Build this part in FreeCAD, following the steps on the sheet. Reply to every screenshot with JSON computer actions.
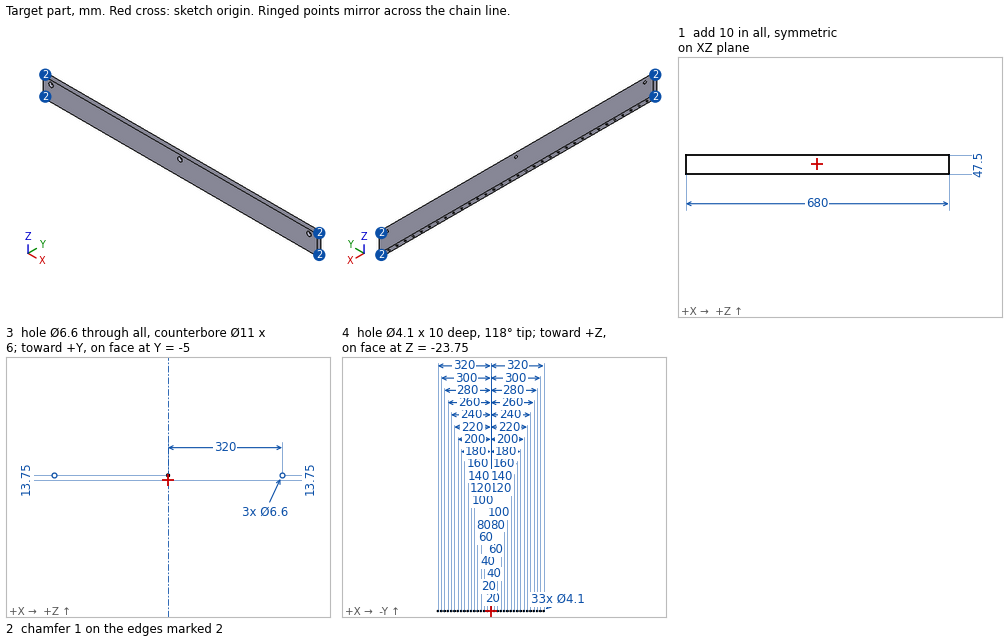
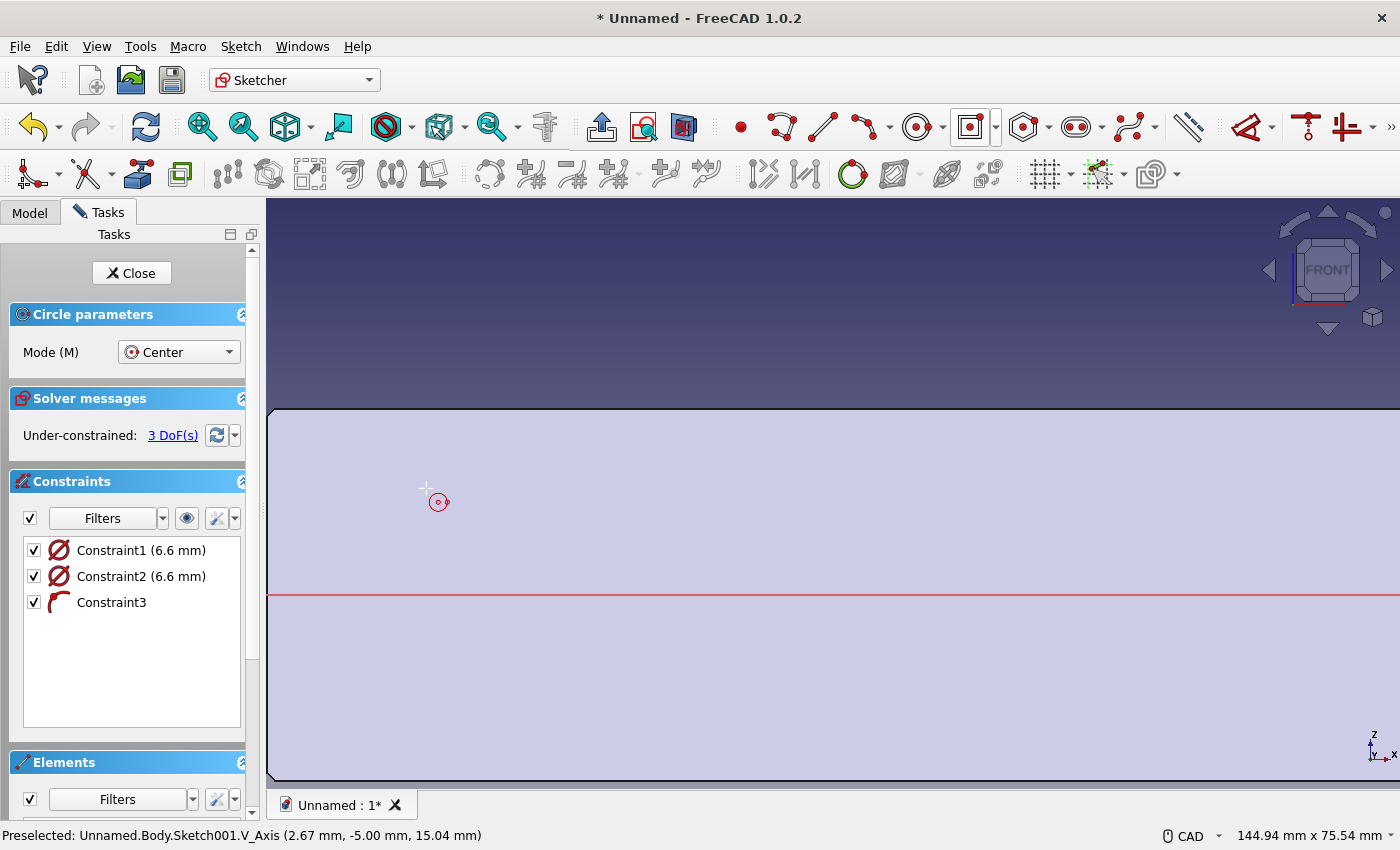
{"action": "scroll", "coordinate": [426, 488], "scroll_direction": "down", "scroll_amount": 10}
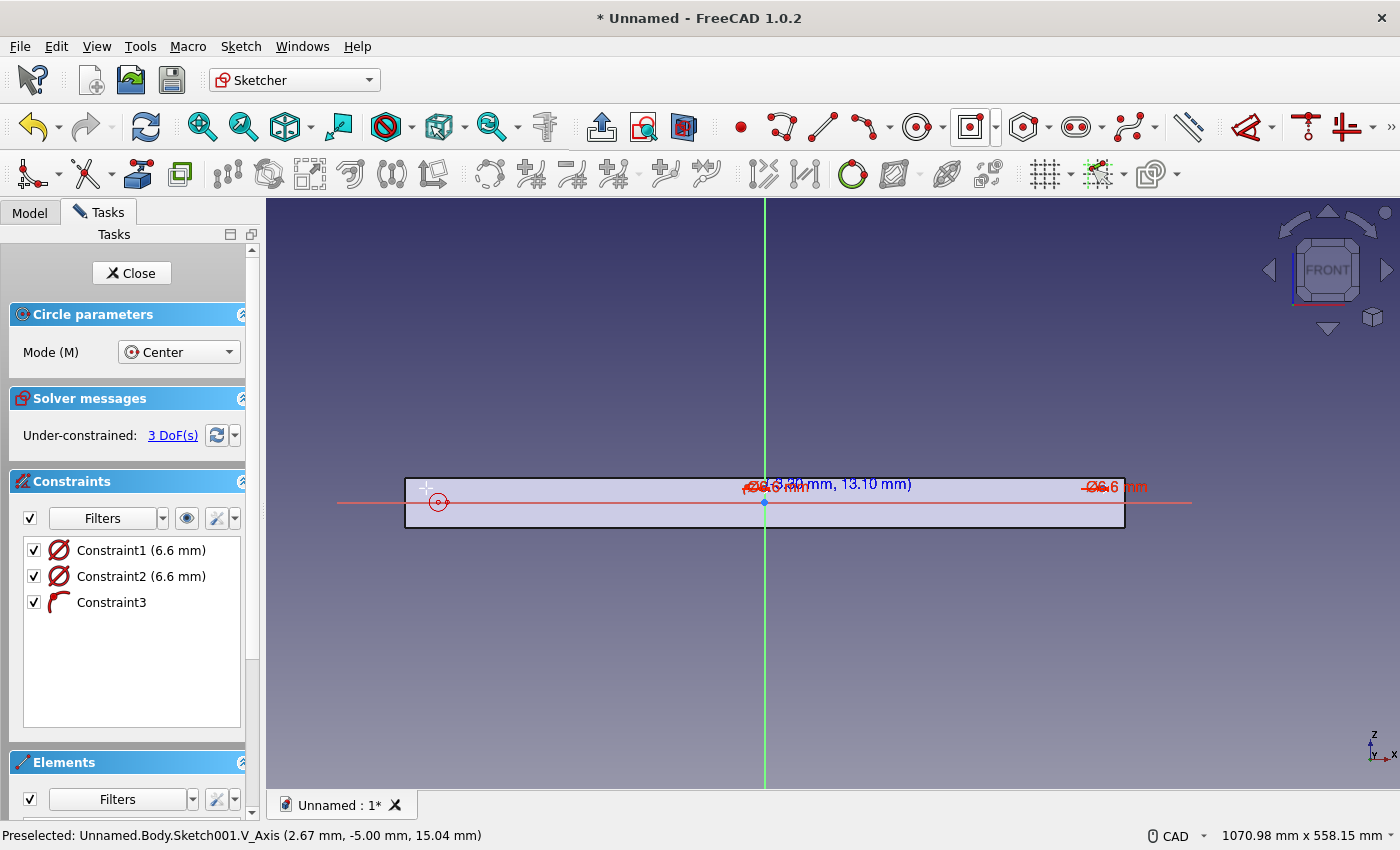
{"action": "left_click", "coordinate": [426, 488]}
{"action": "mouse_move", "coordinate": [428, 486]}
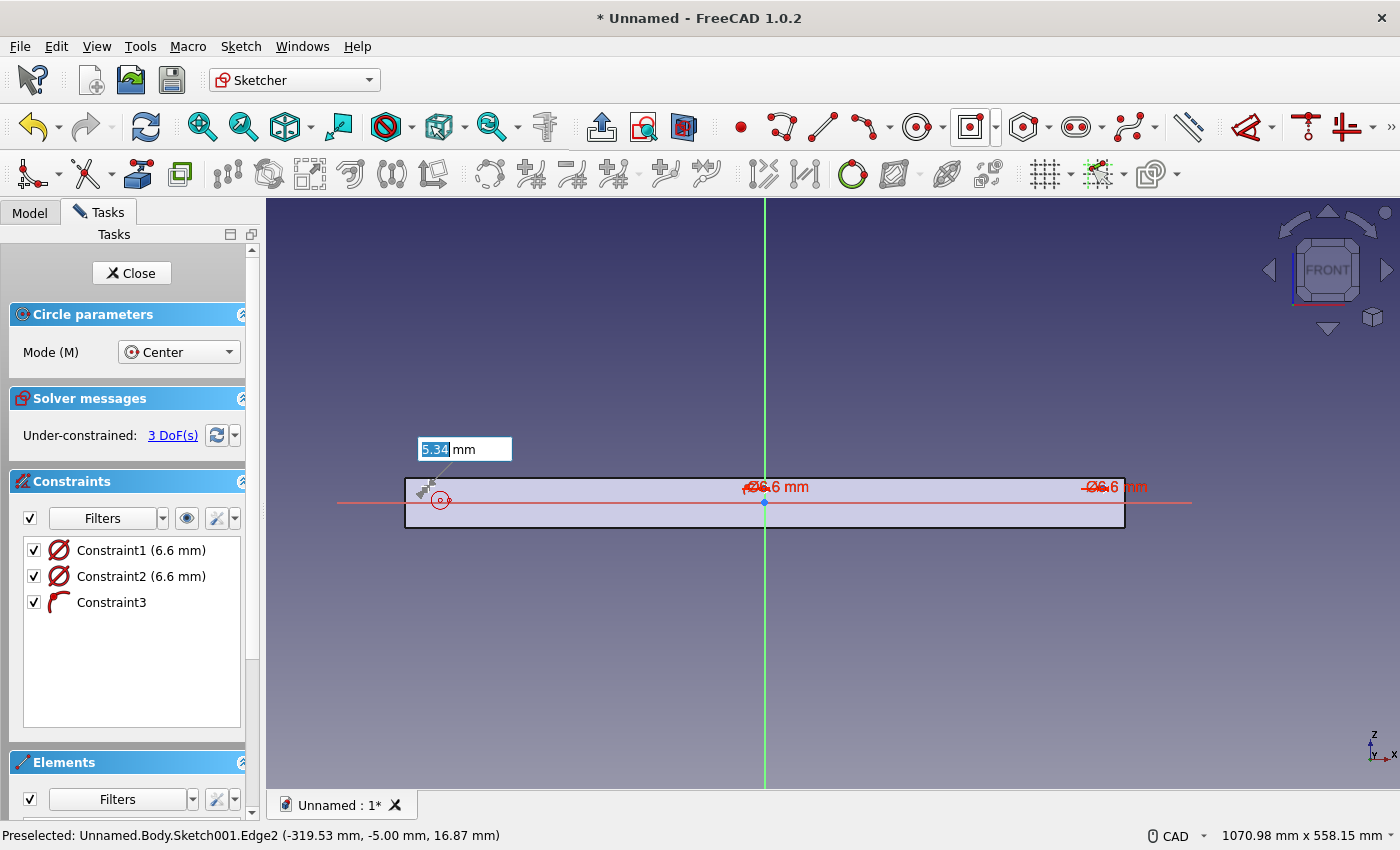
{"action": "type", "text": "6.6"}
{"action": "key", "text": "Return"}
{"action": "key", "text": "Escape"}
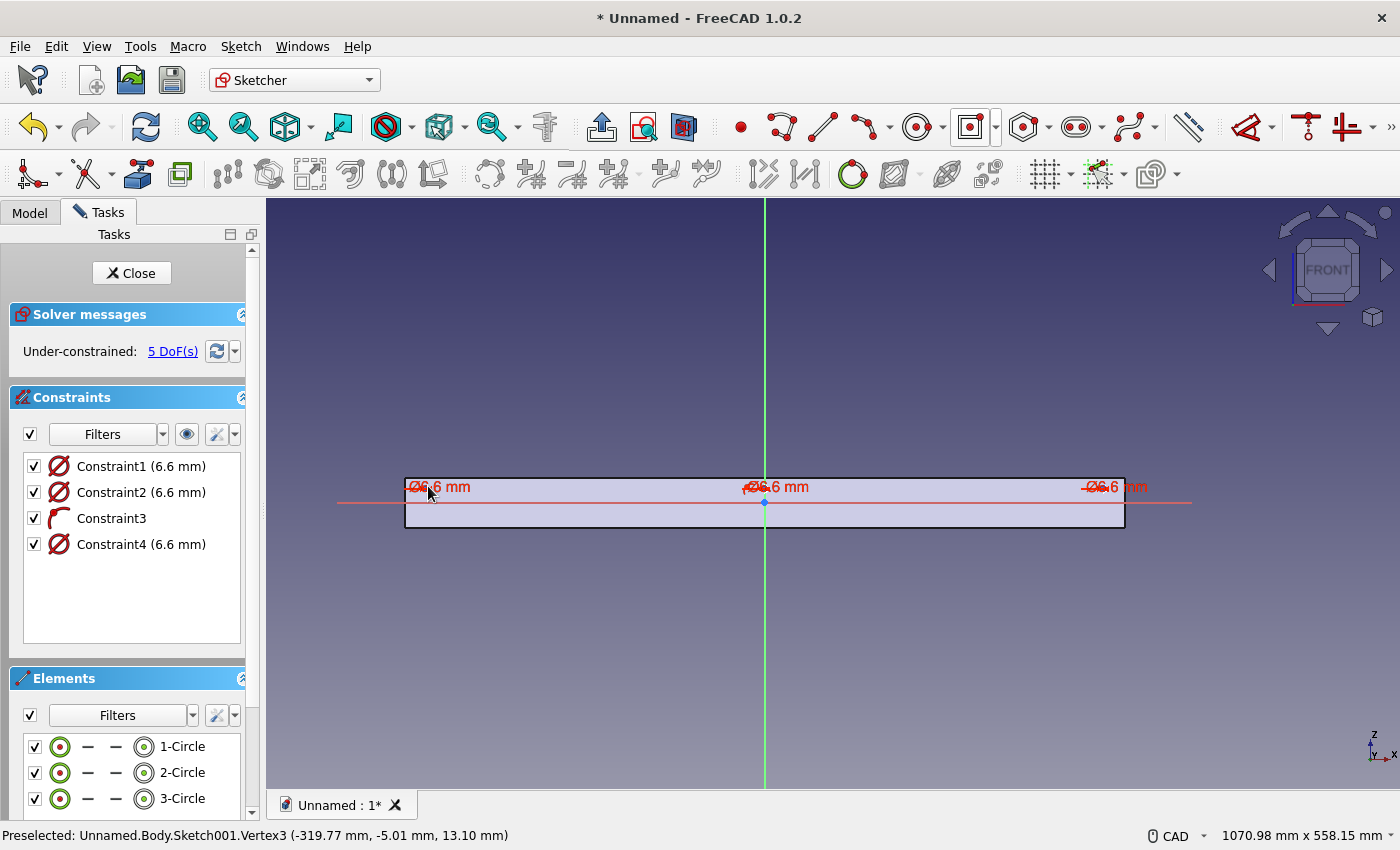
{"action": "left_click", "coordinate": [1103, 489]}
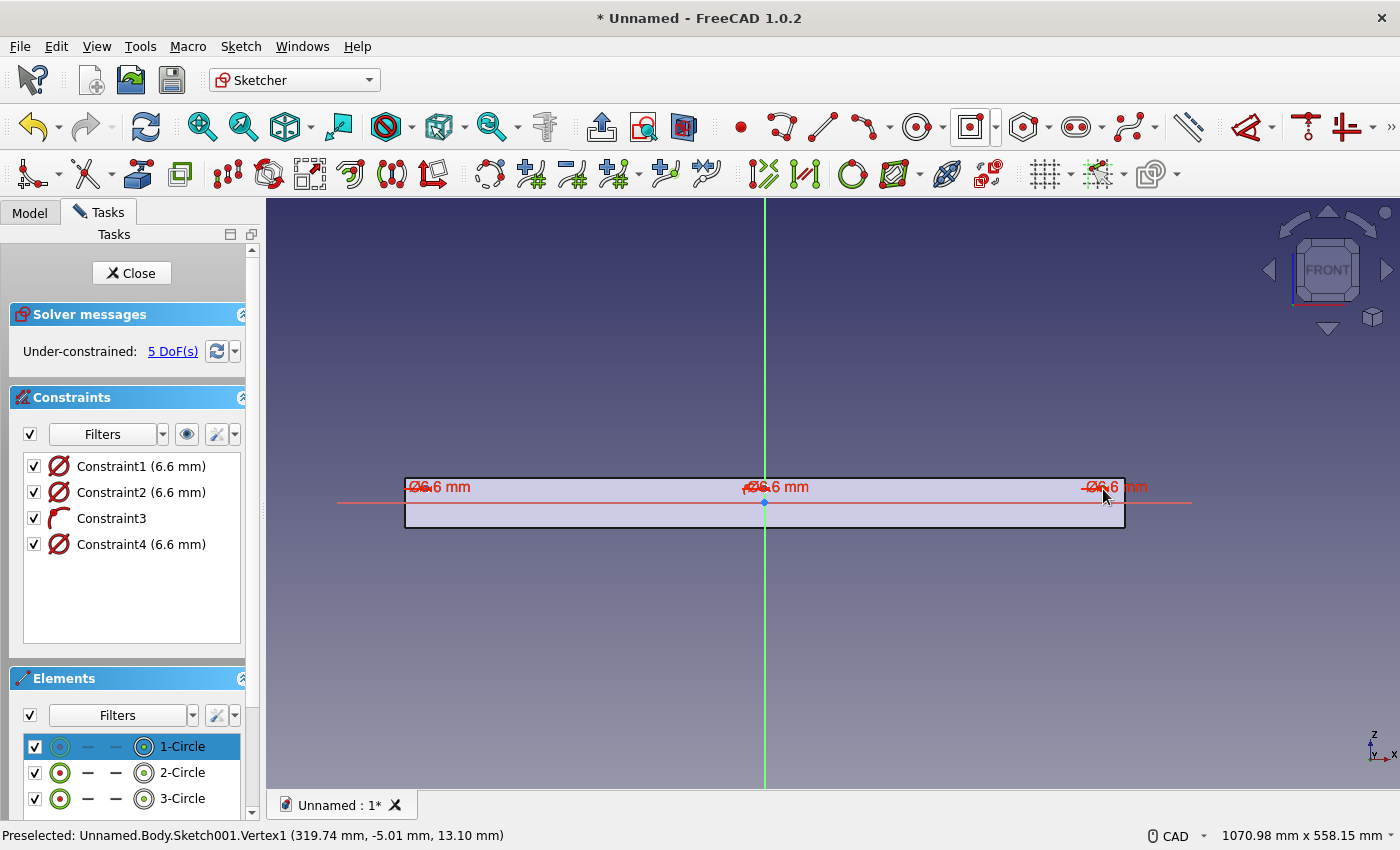
{"action": "left_click", "coordinate": [426, 489]}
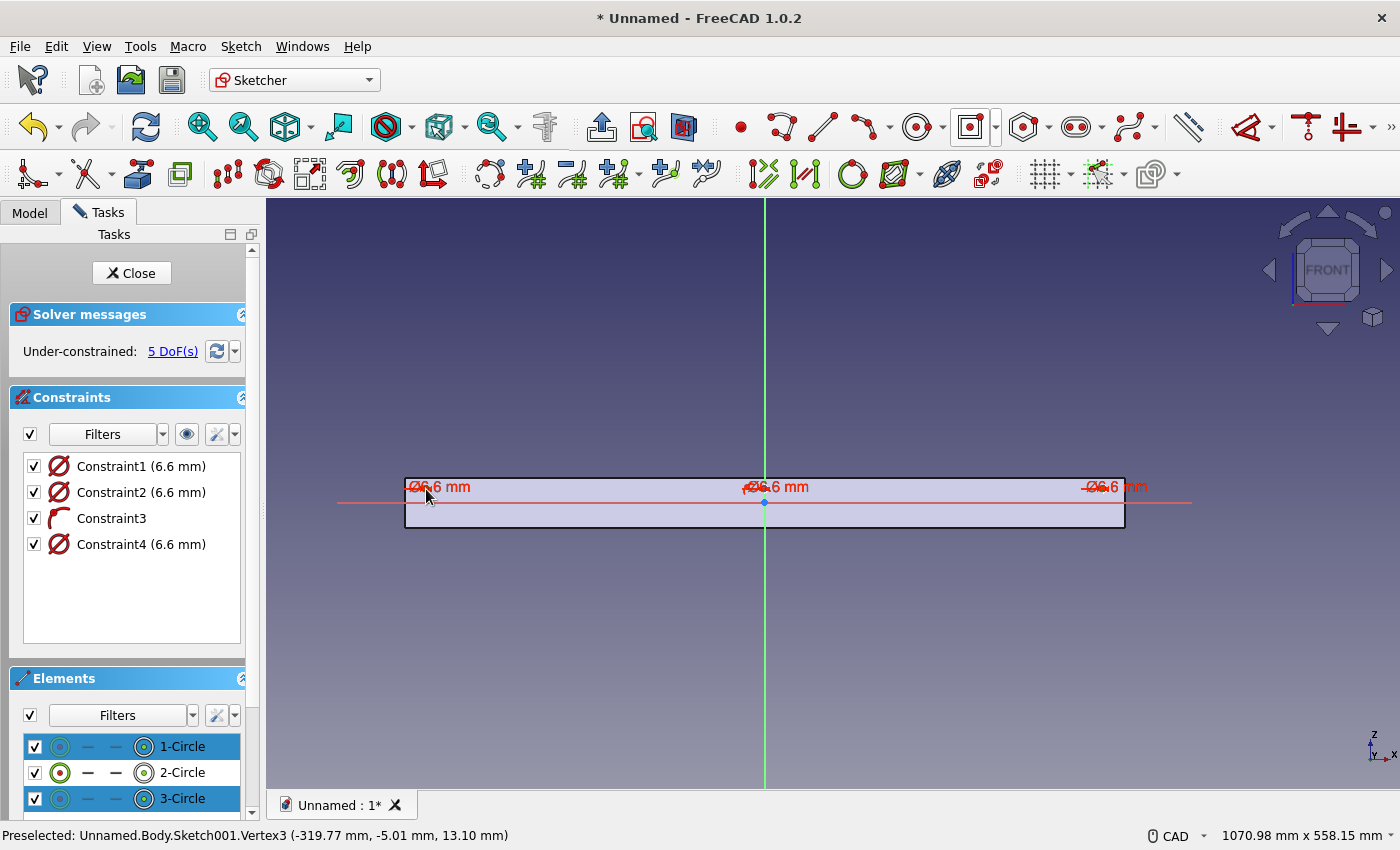
{"action": "left_click", "coordinate": [765, 723]}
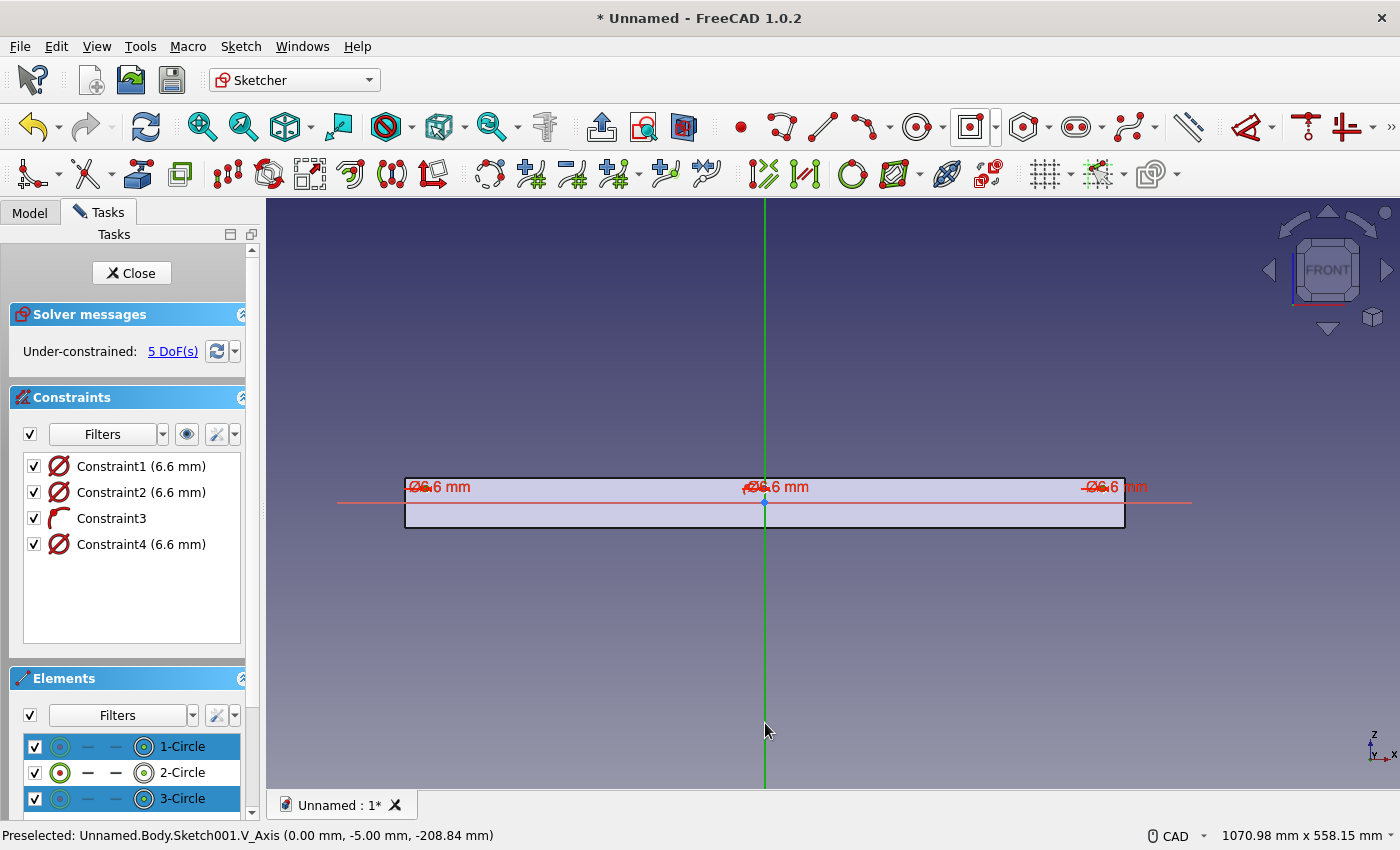
{"action": "key", "text": "s"}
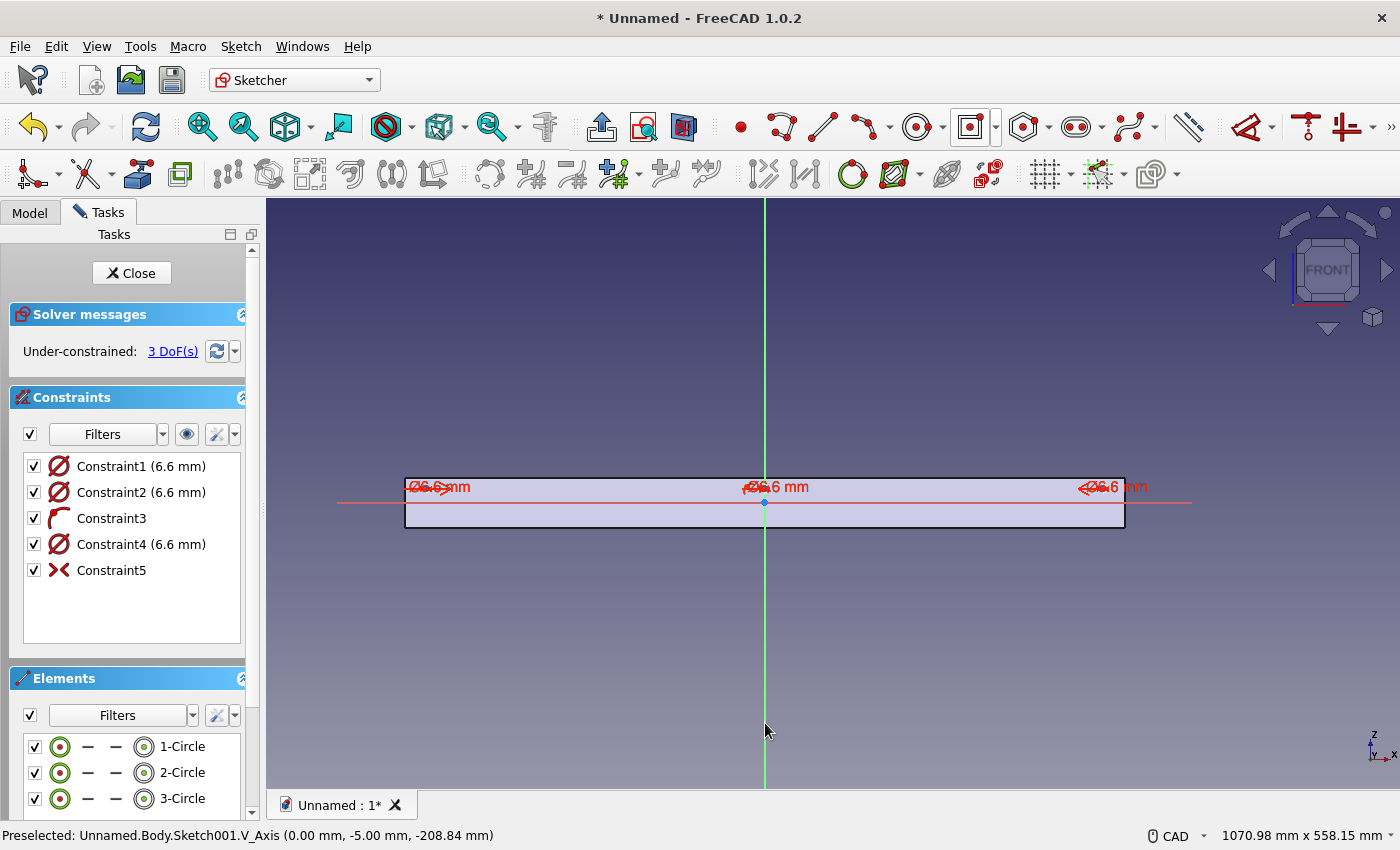
{"action": "left_click", "coordinate": [1246, 128]}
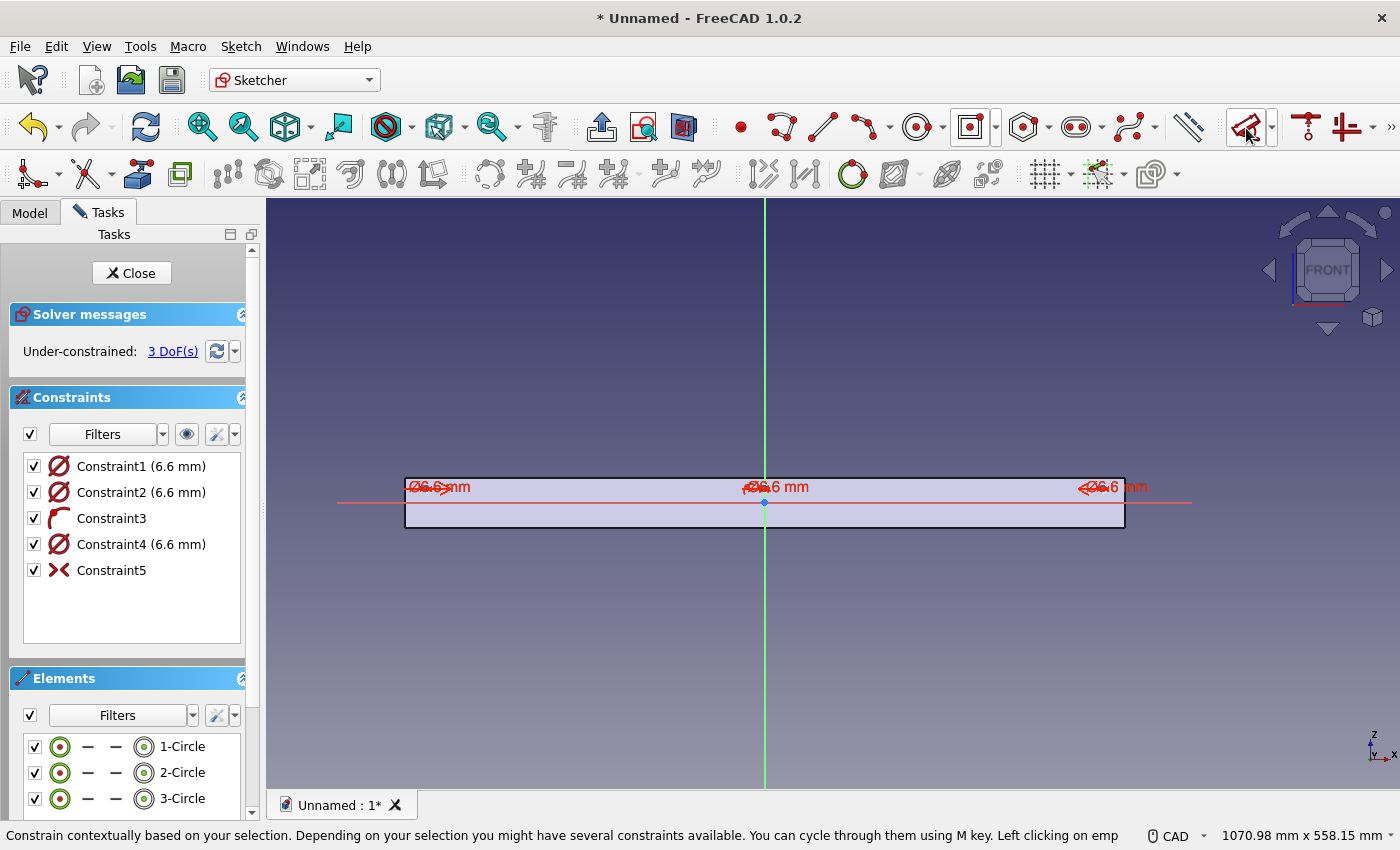
{"action": "left_click", "coordinate": [1103, 489]}
{"action": "left_click", "coordinate": [934, 537]}